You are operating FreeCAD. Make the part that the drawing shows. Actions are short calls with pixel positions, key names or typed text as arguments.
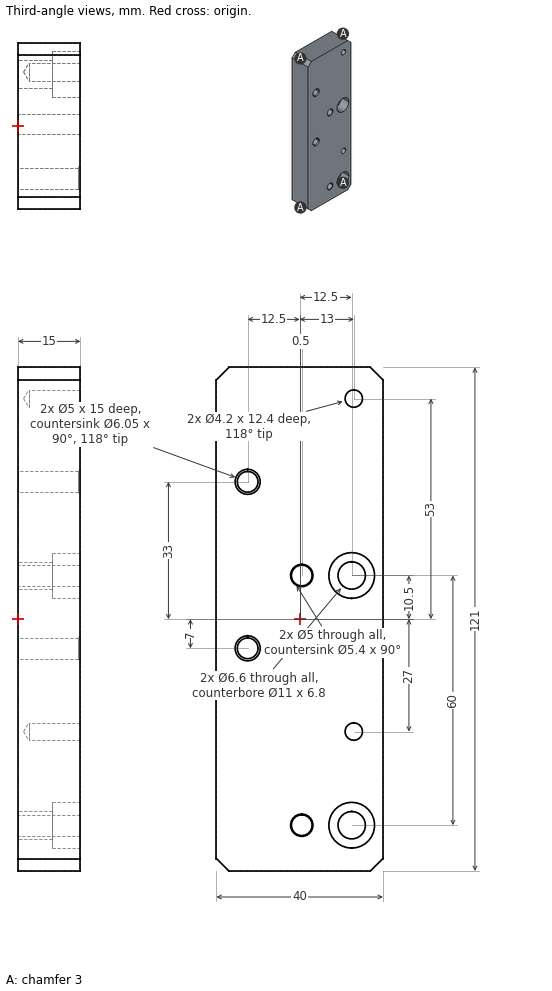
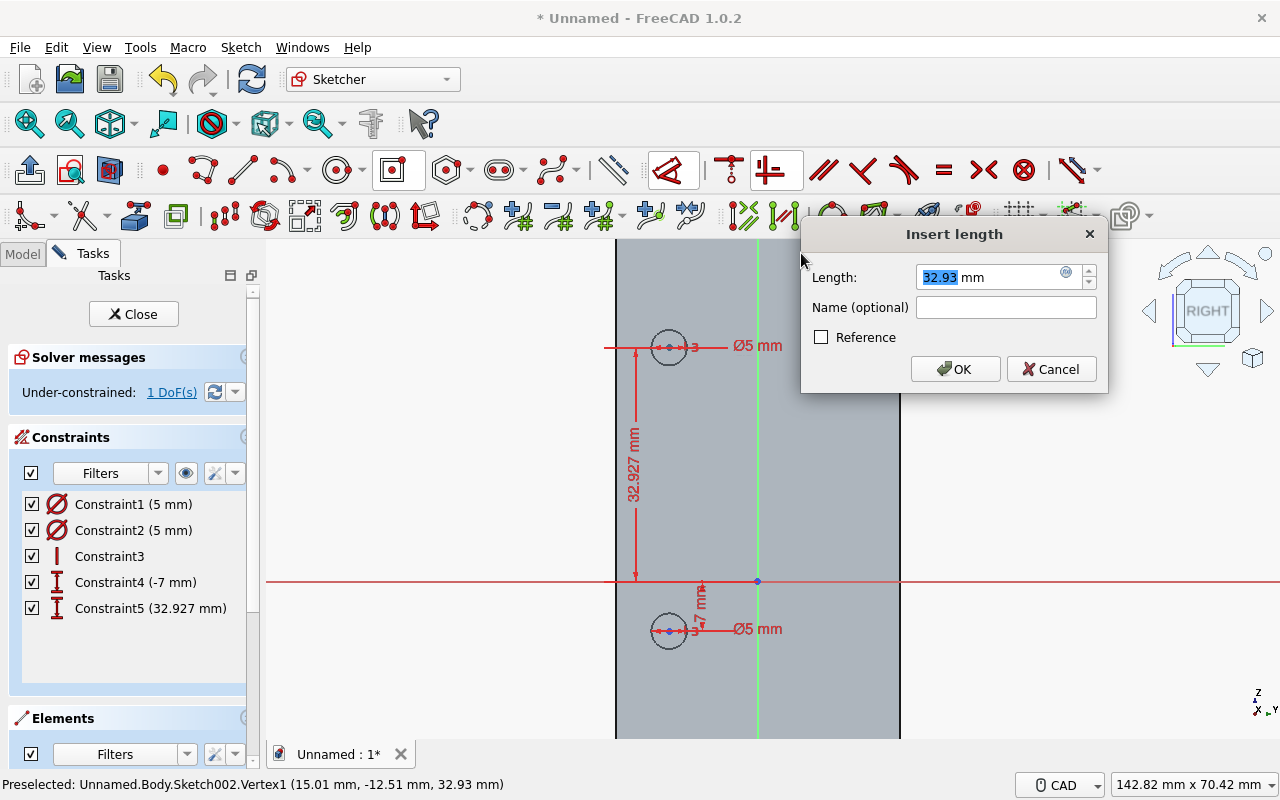
text(33)
key(Return)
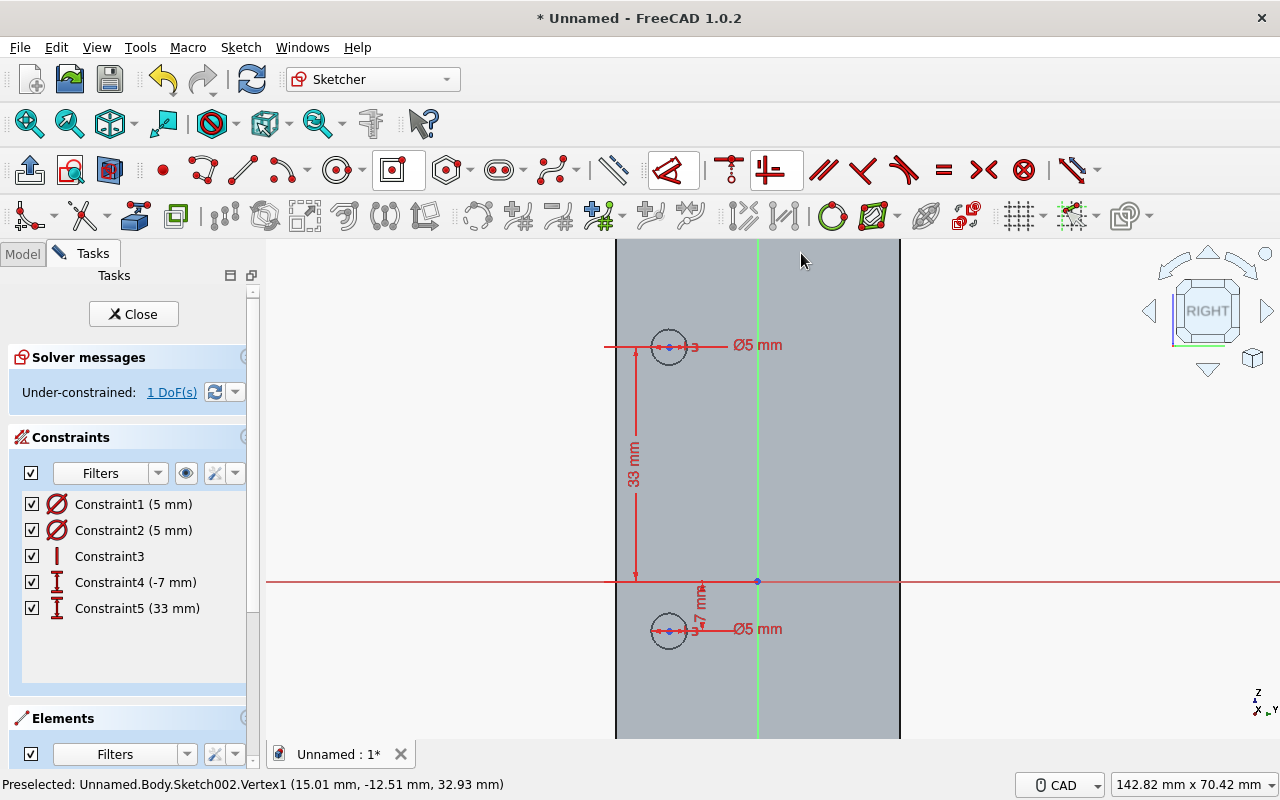
click(669, 347)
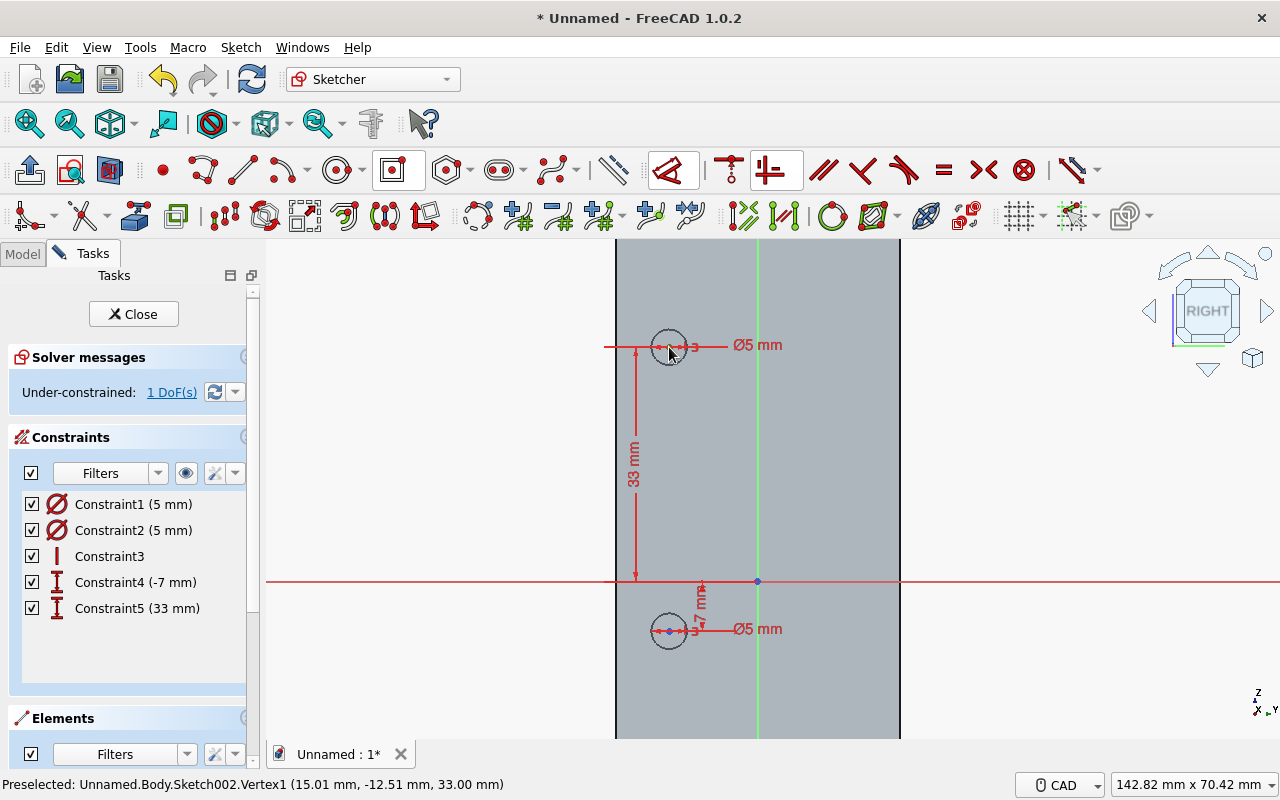
click(694, 170)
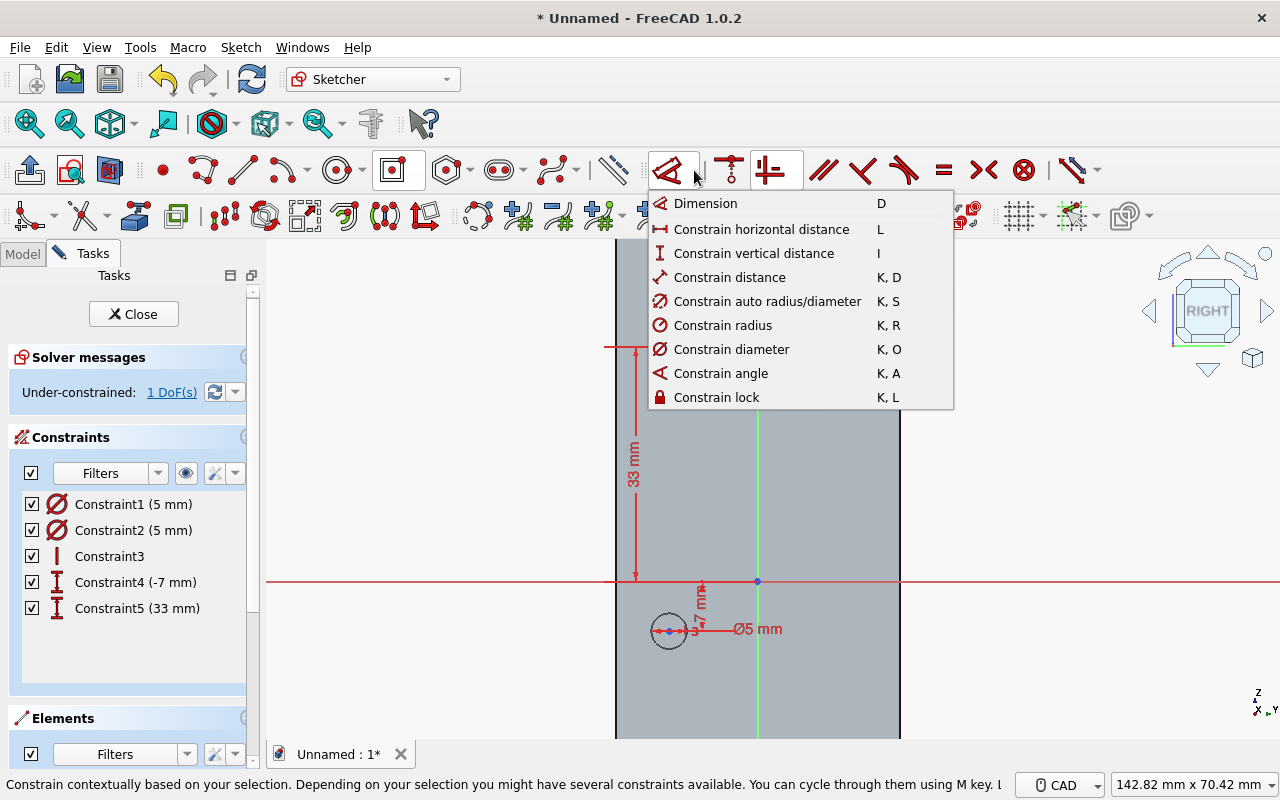
click(801, 229)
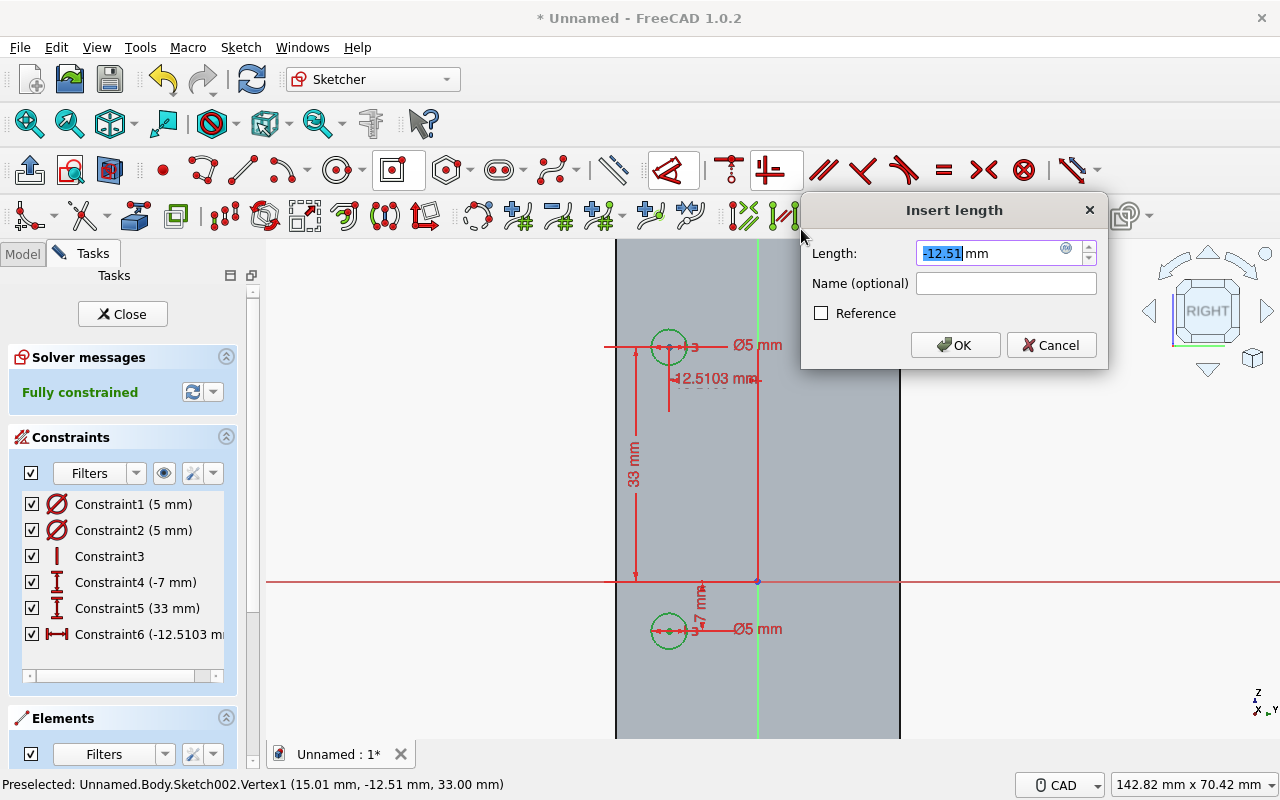
text(-12.5)
key(Return)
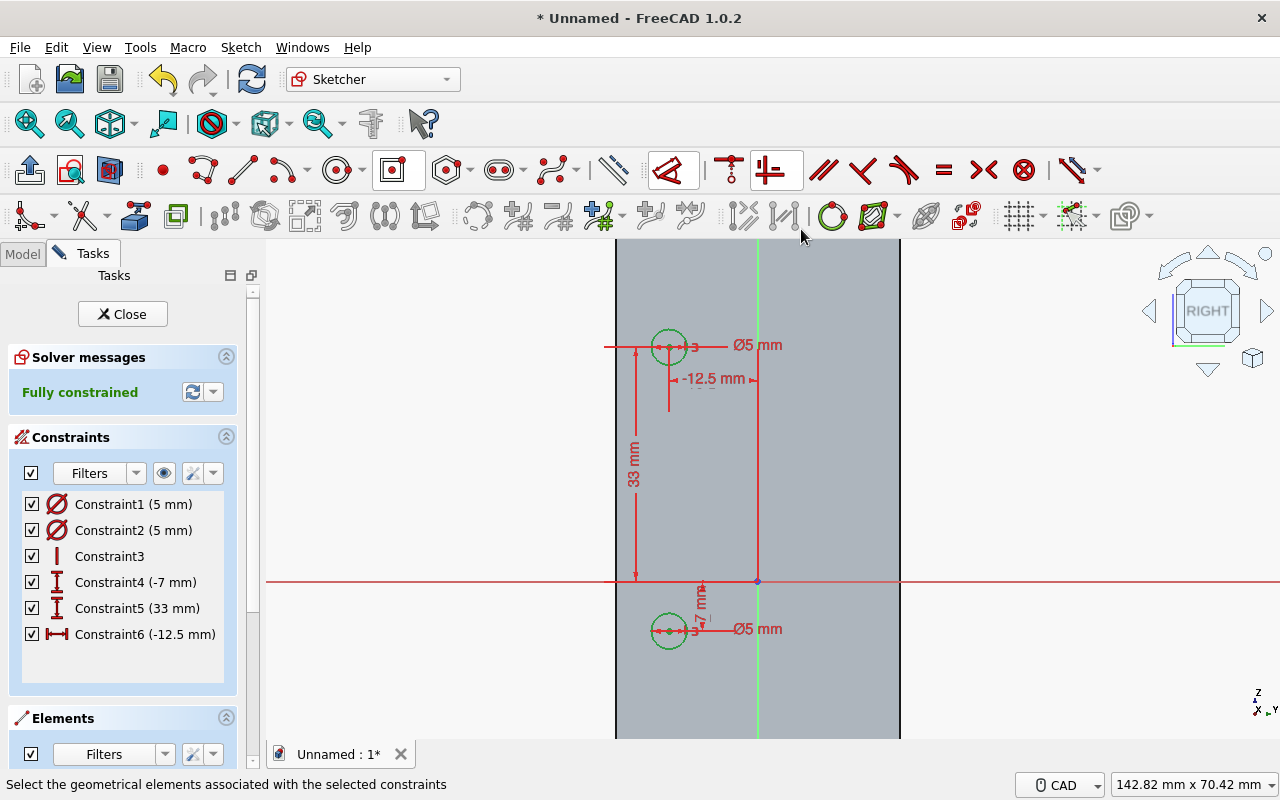
click(123, 314)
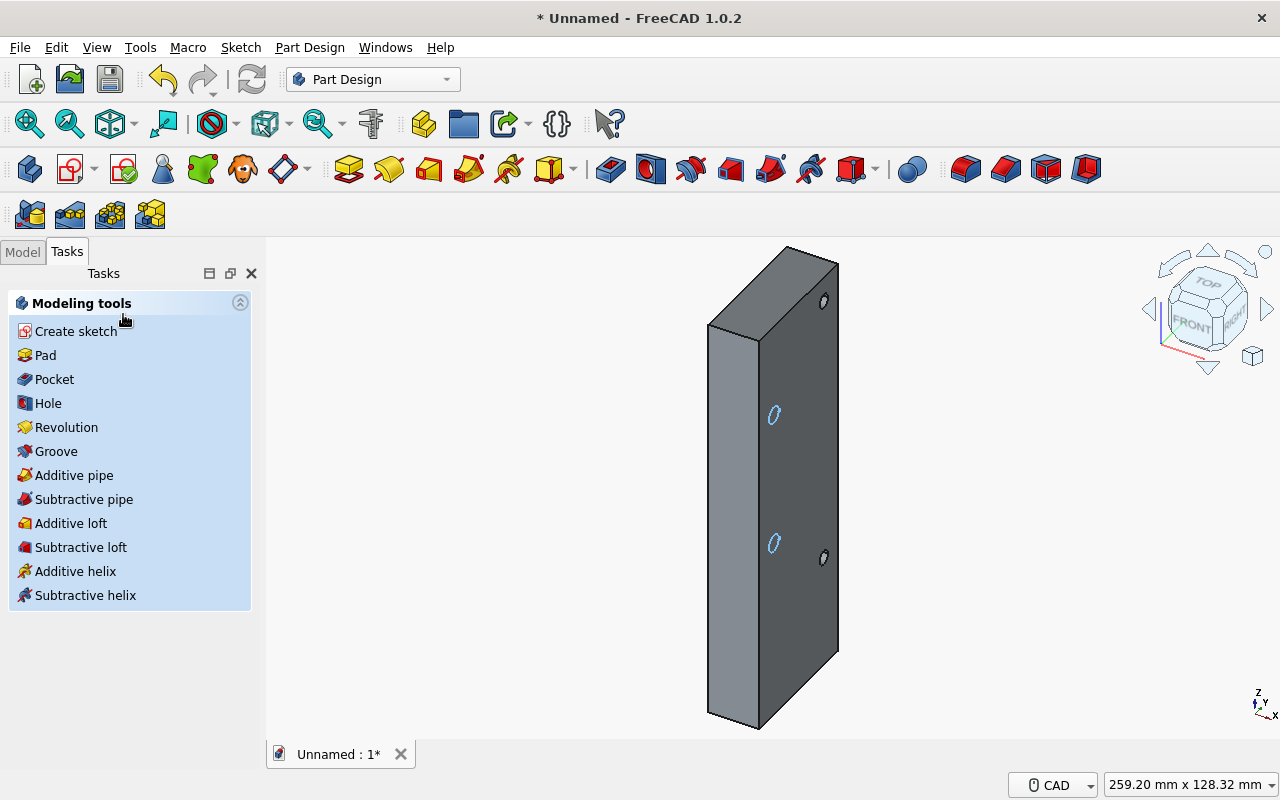
click(652, 170)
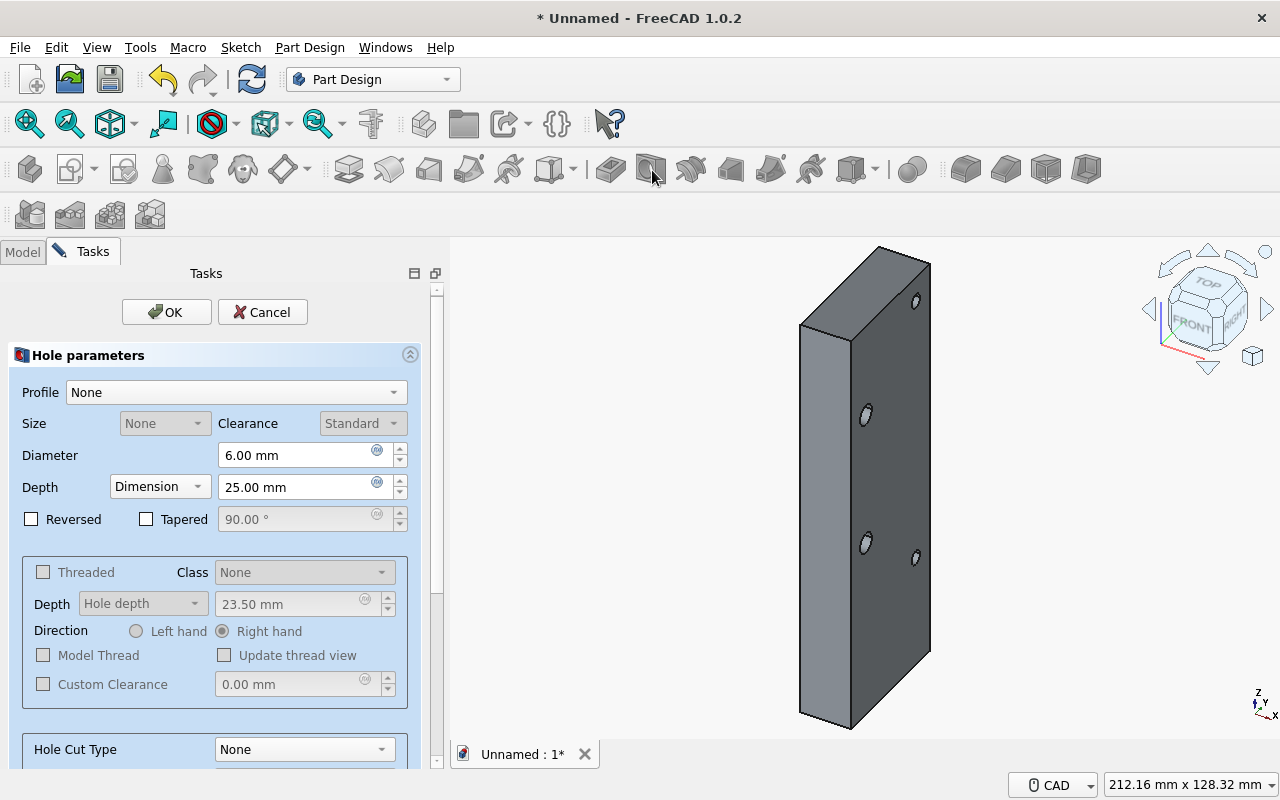
triple_click(305, 455)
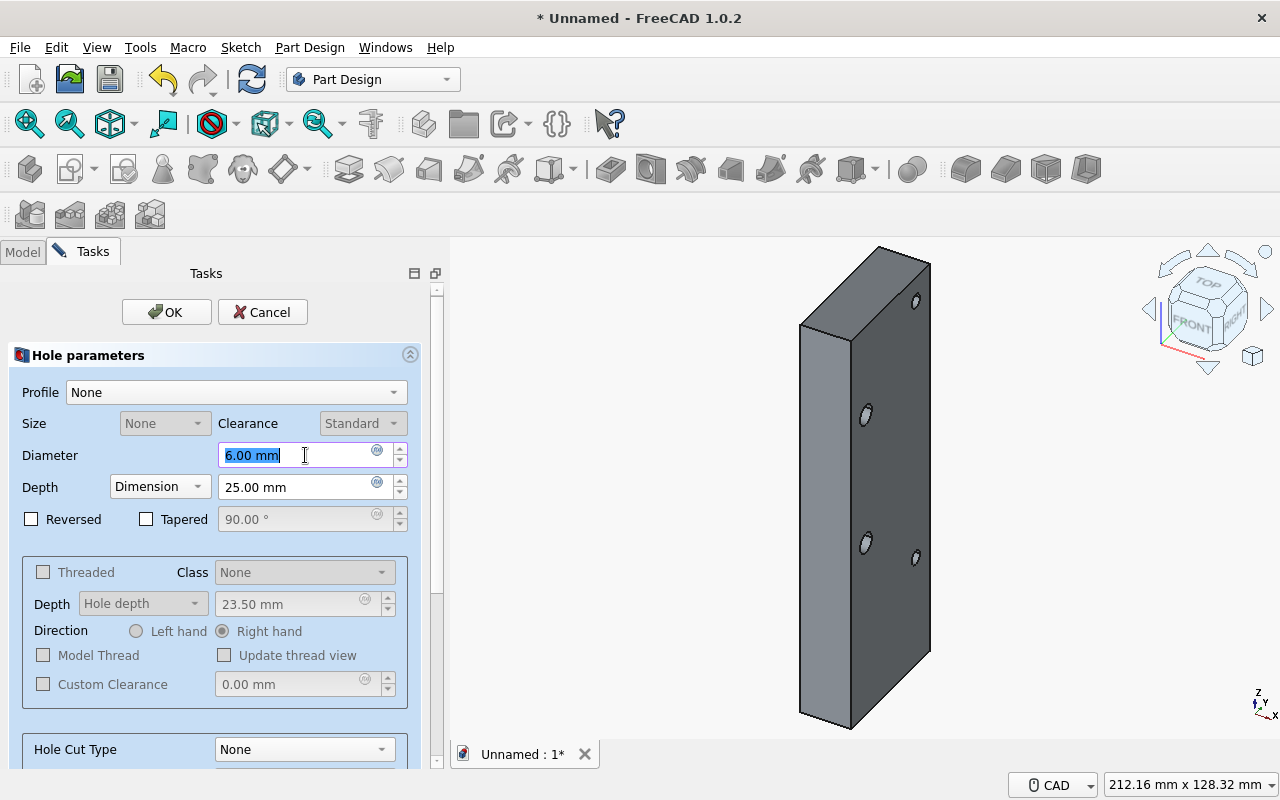
text(5)
key(Tab)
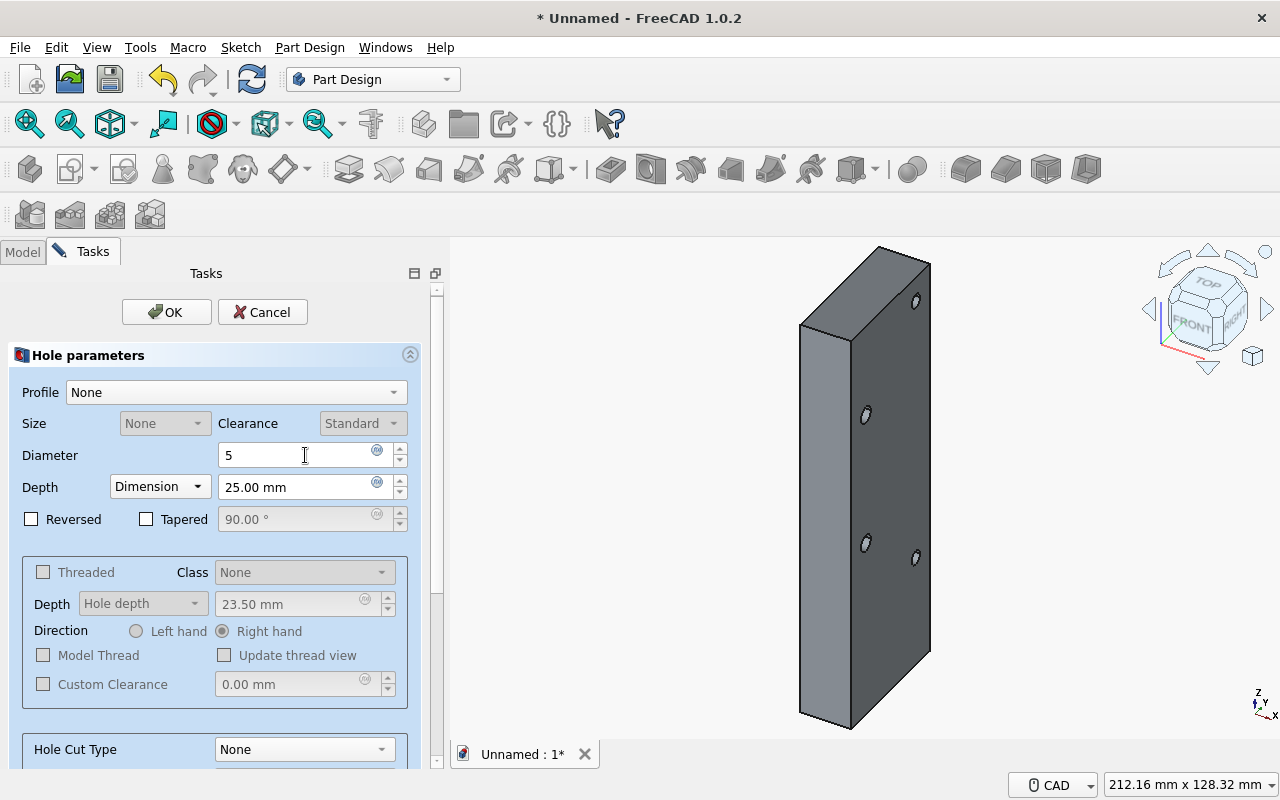
triple_click(305, 487)